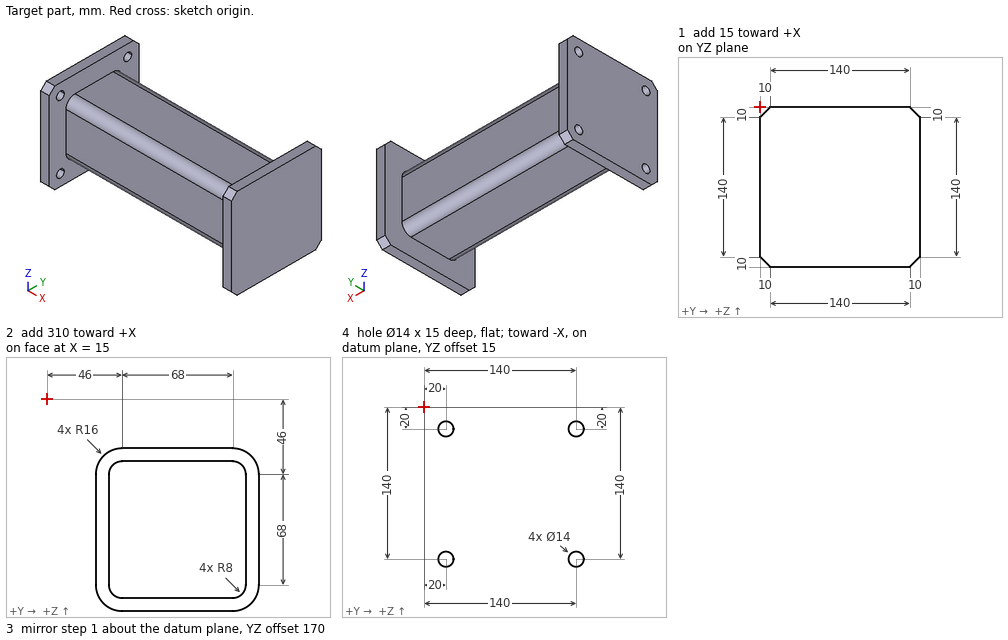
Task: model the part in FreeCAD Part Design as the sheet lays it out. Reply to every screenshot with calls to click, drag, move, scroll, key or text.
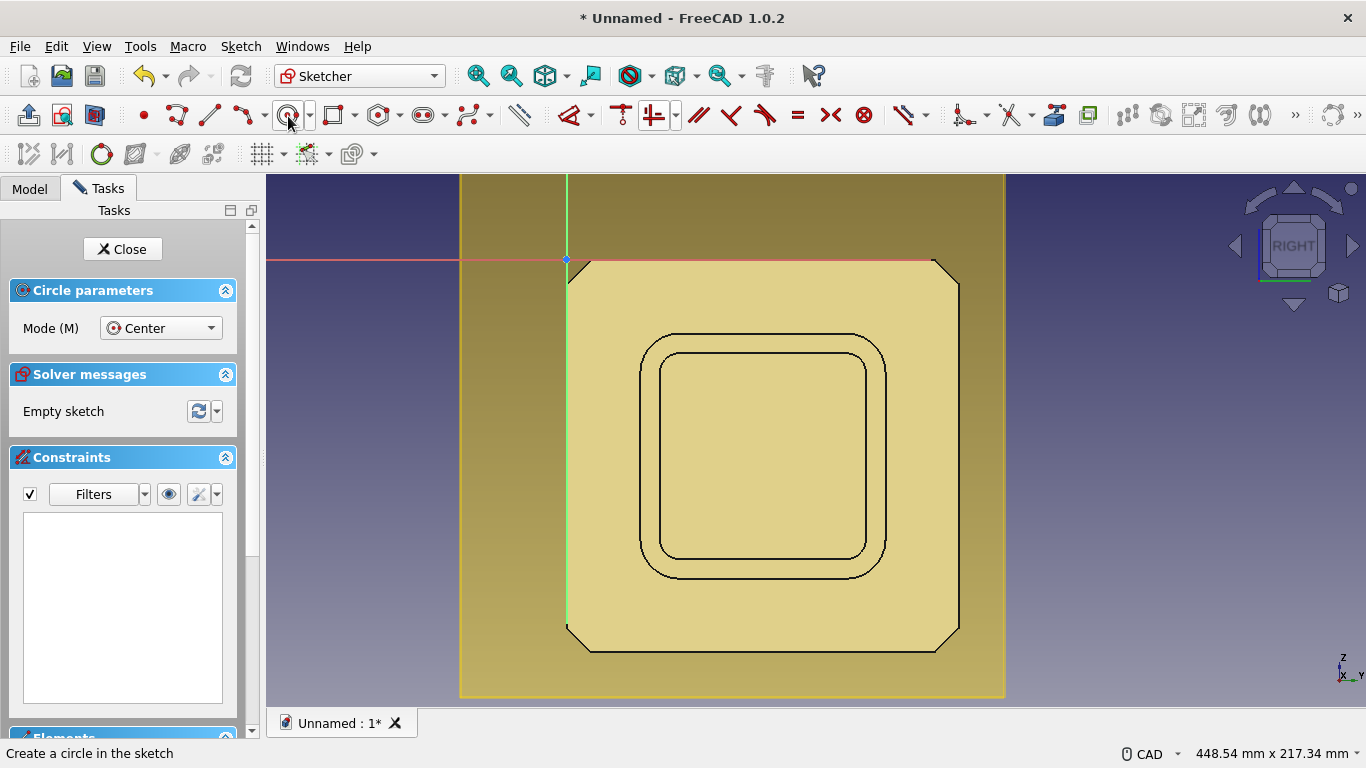
scroll(910, 603, up, 2)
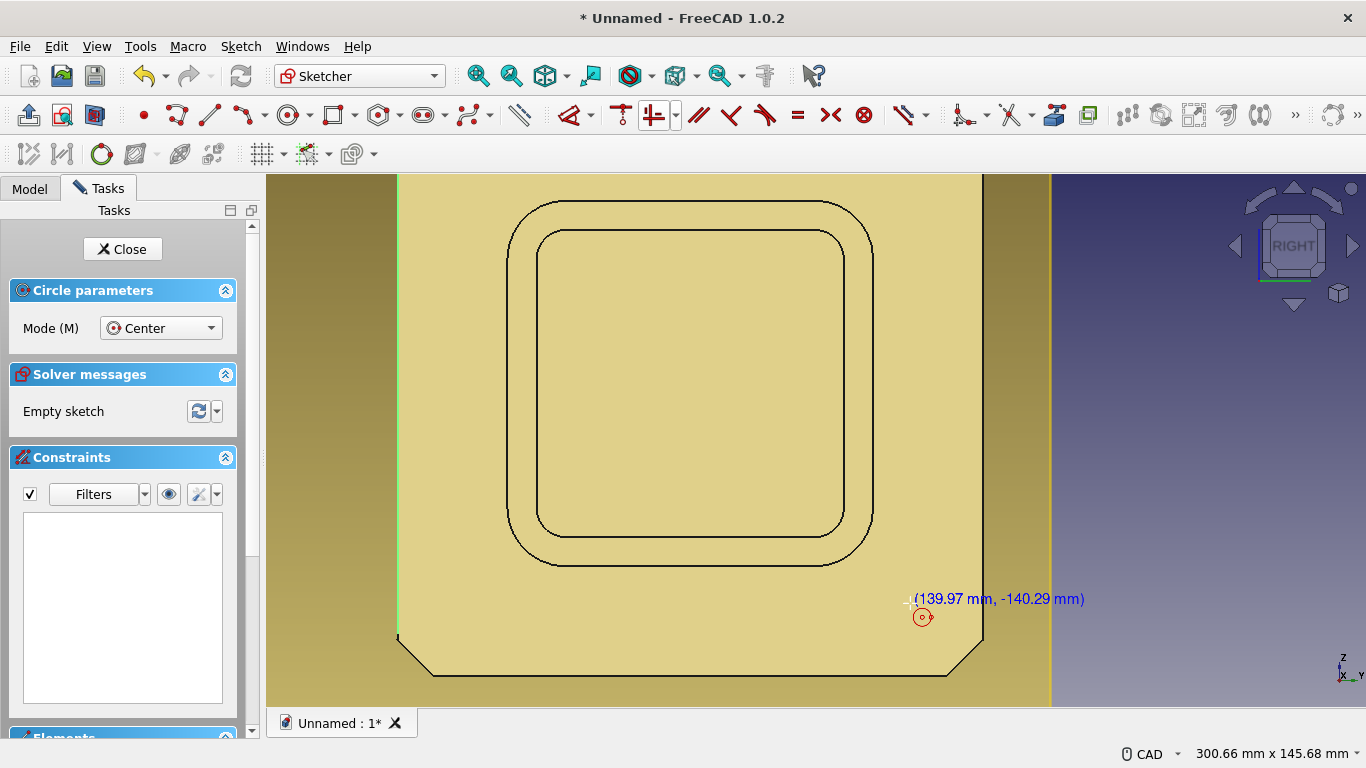
click(910, 603)
move(928, 585)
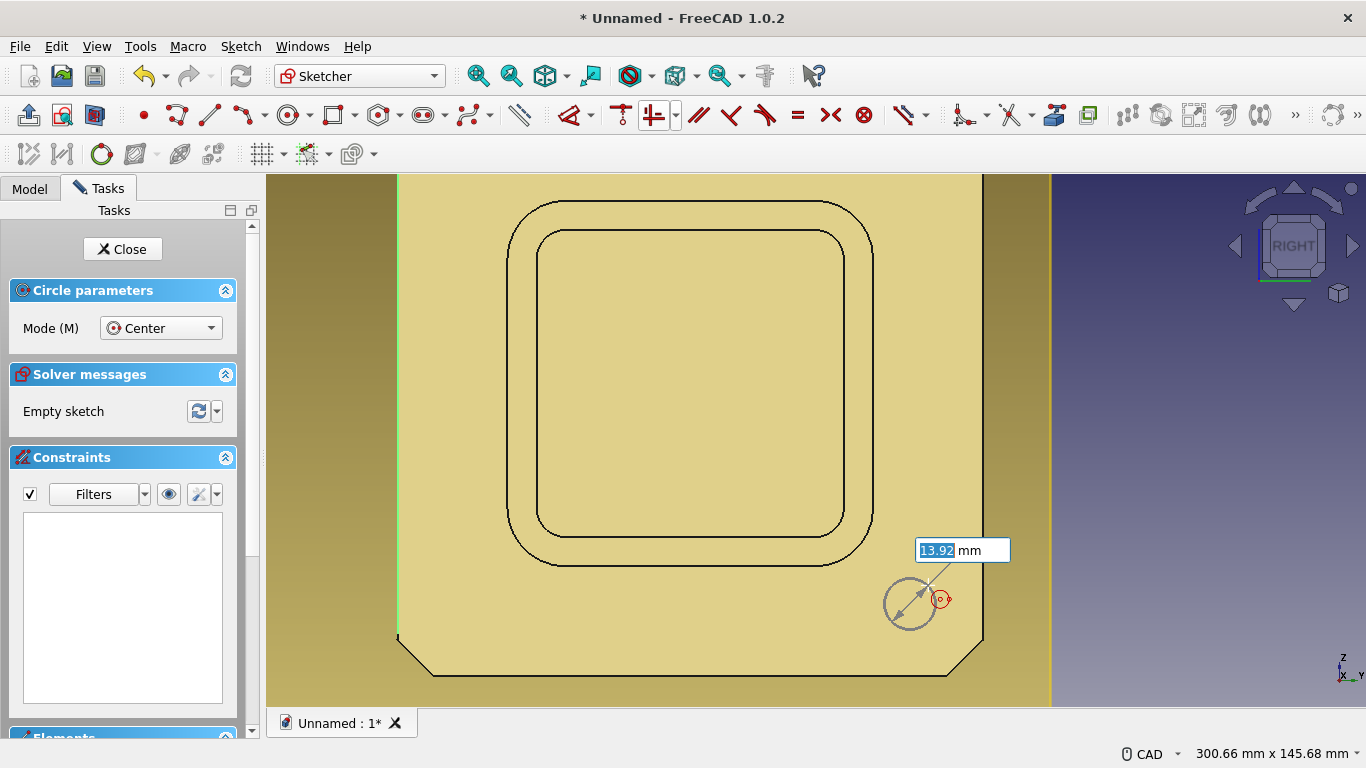
text(14)
key(Return)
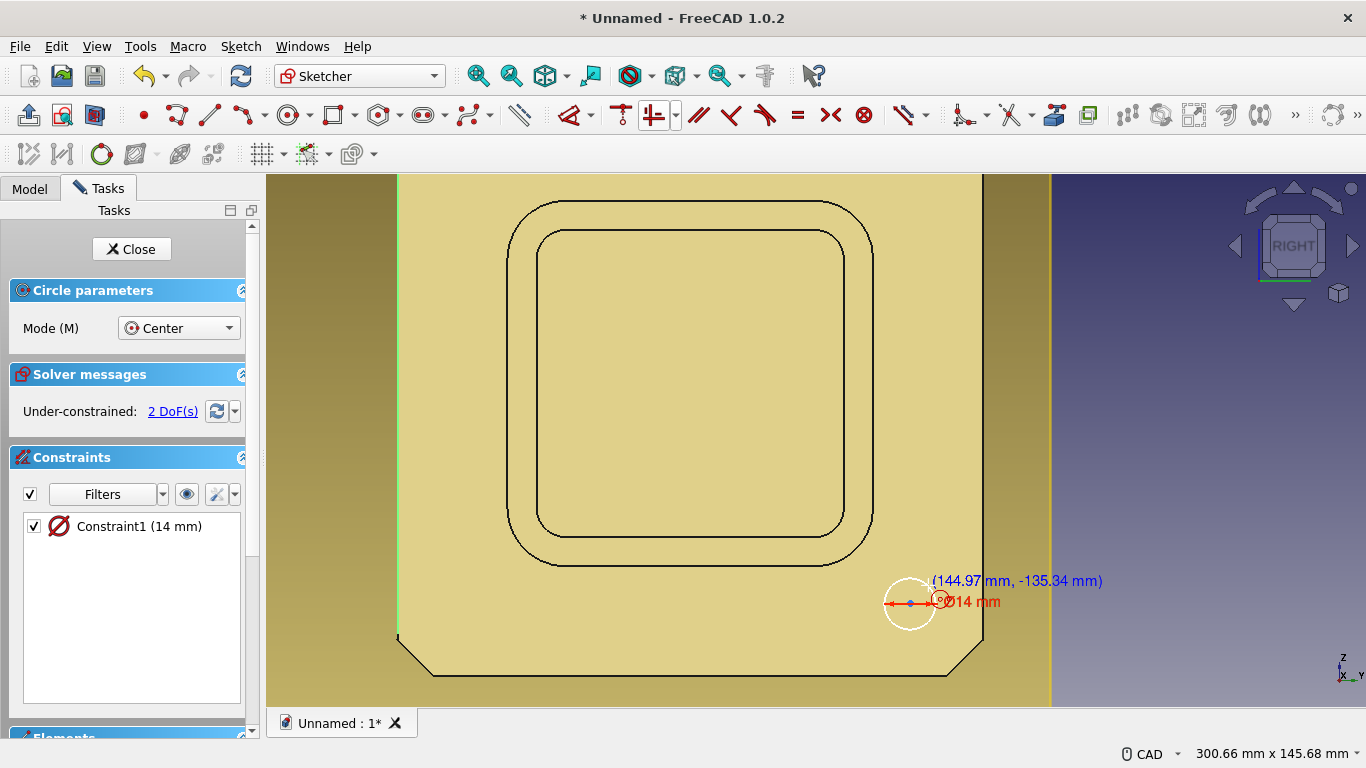
click(471, 603)
move(489, 585)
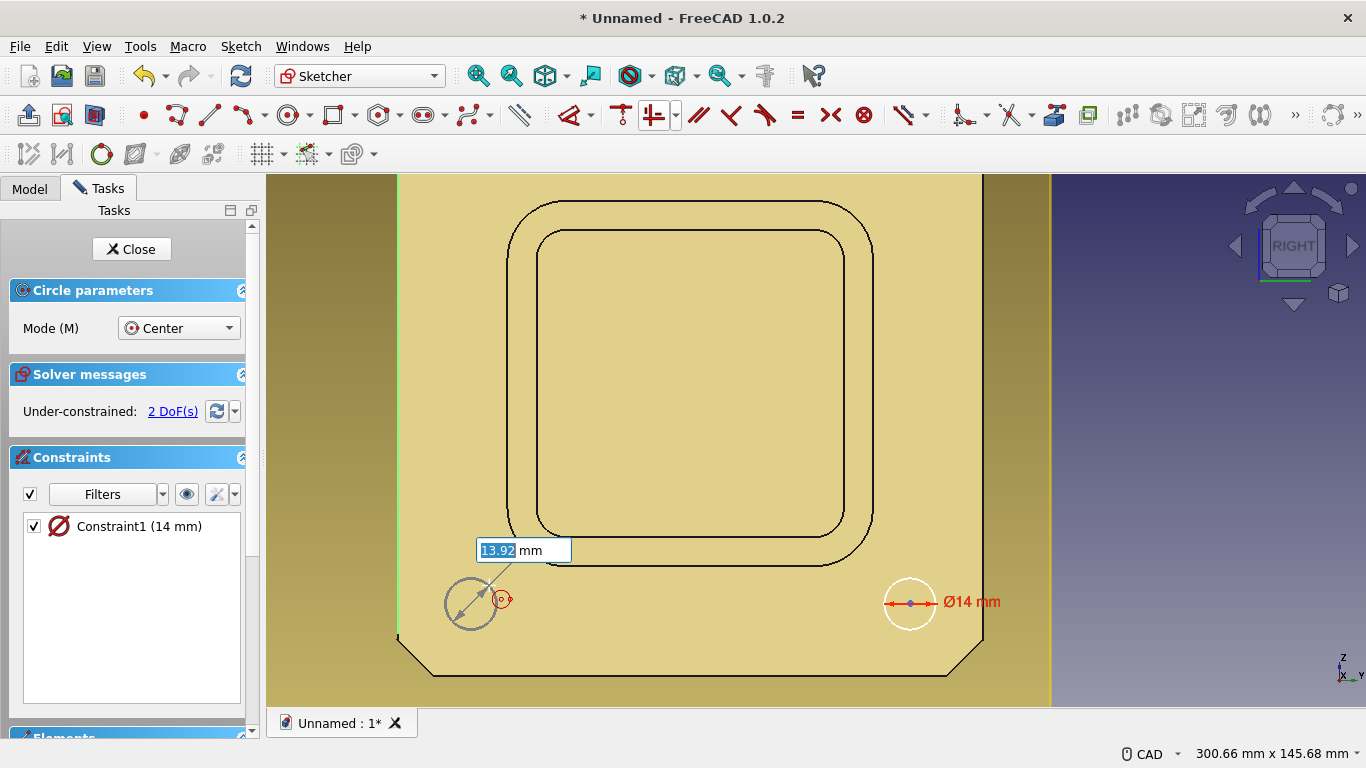
text(14)
key(Return)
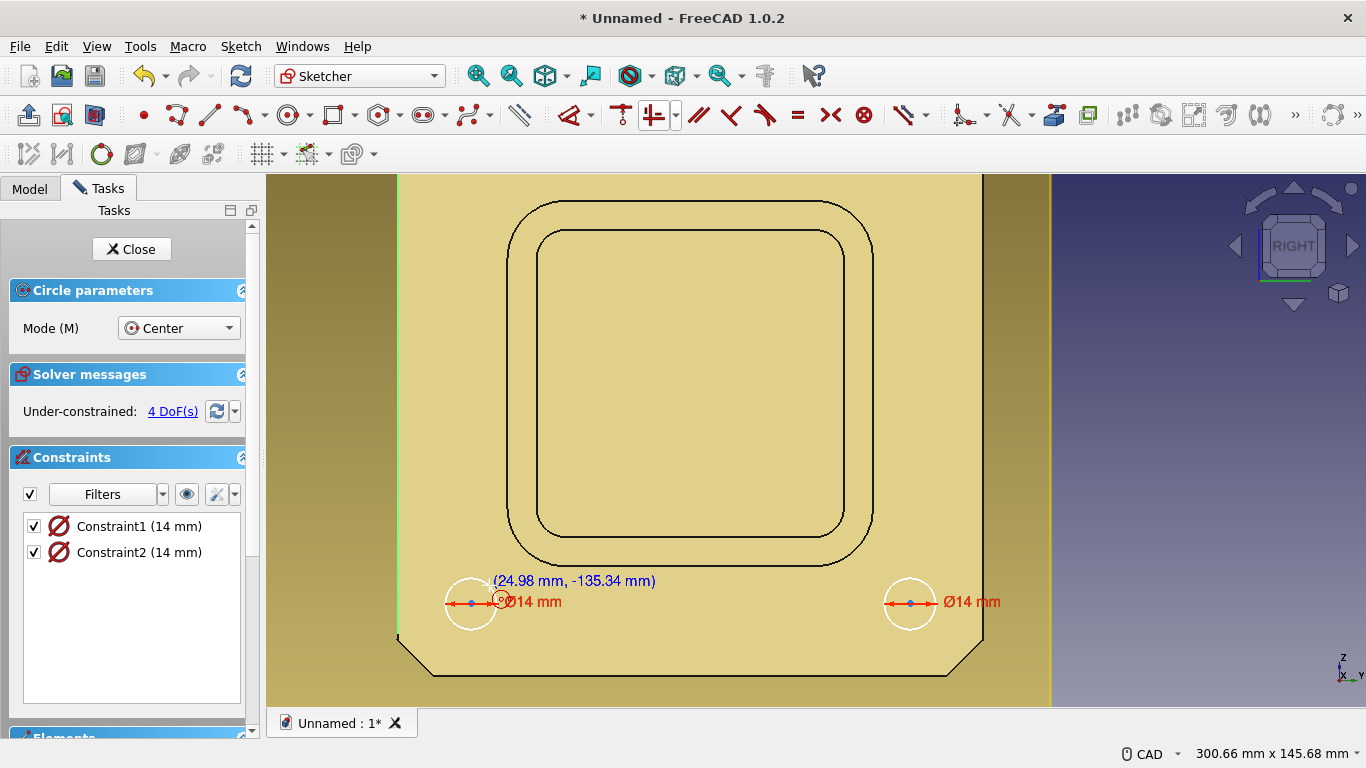
scroll(912, 605, down, 2)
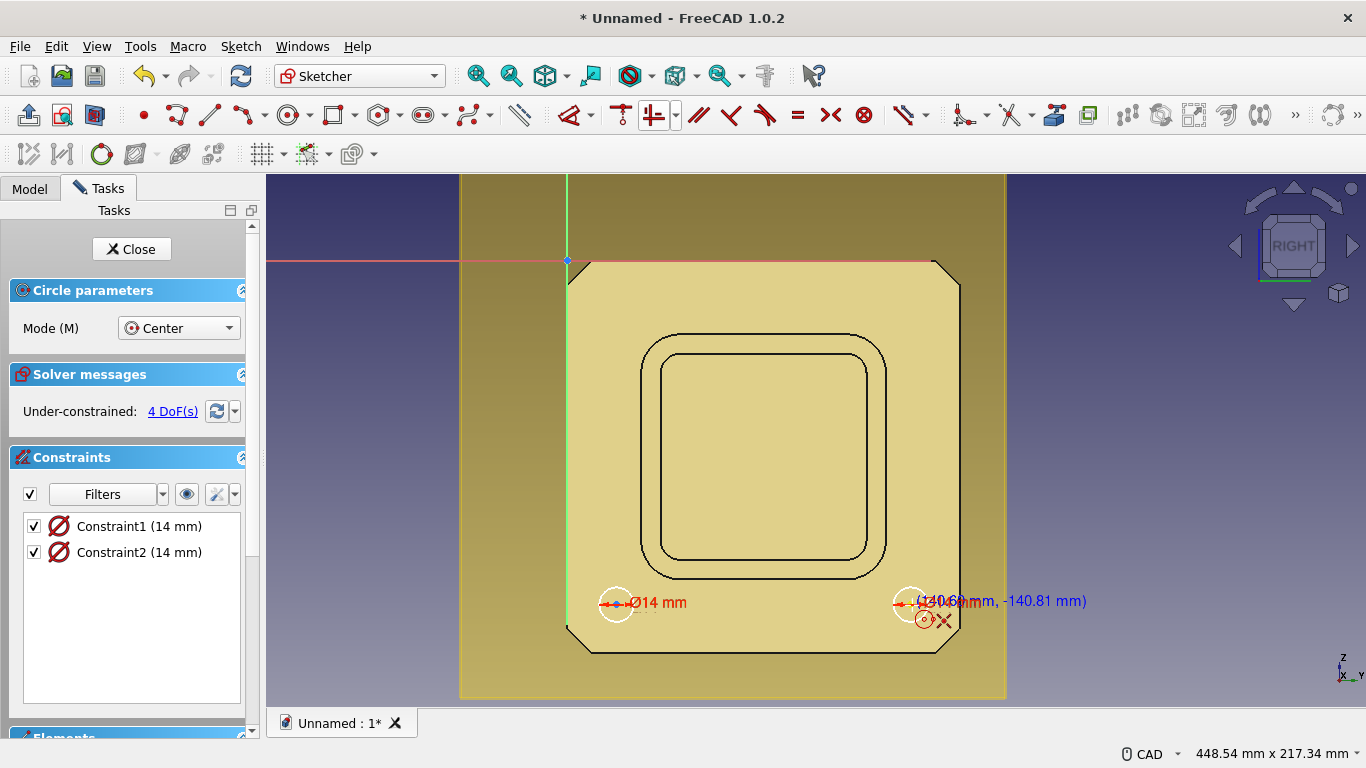
scroll(911, 310, up, 2)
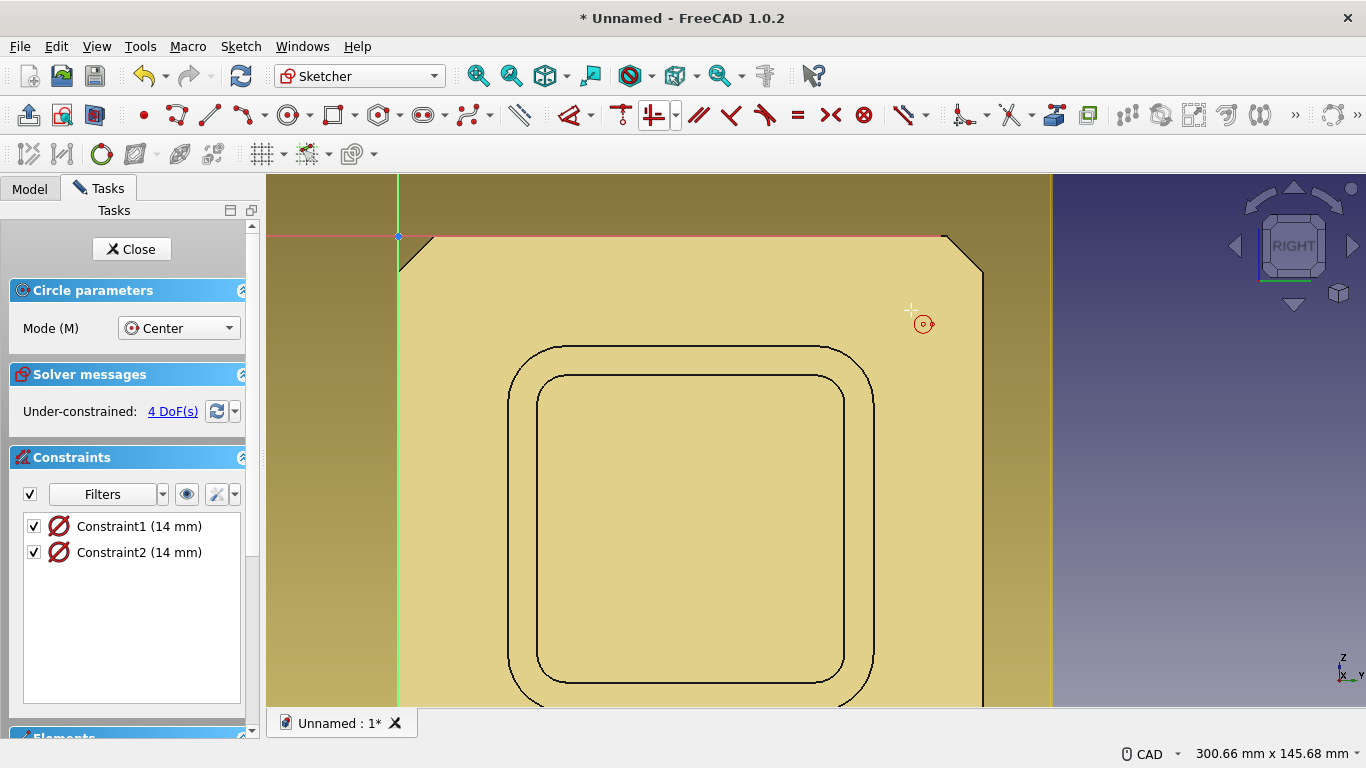
click(910, 309)
move(928, 291)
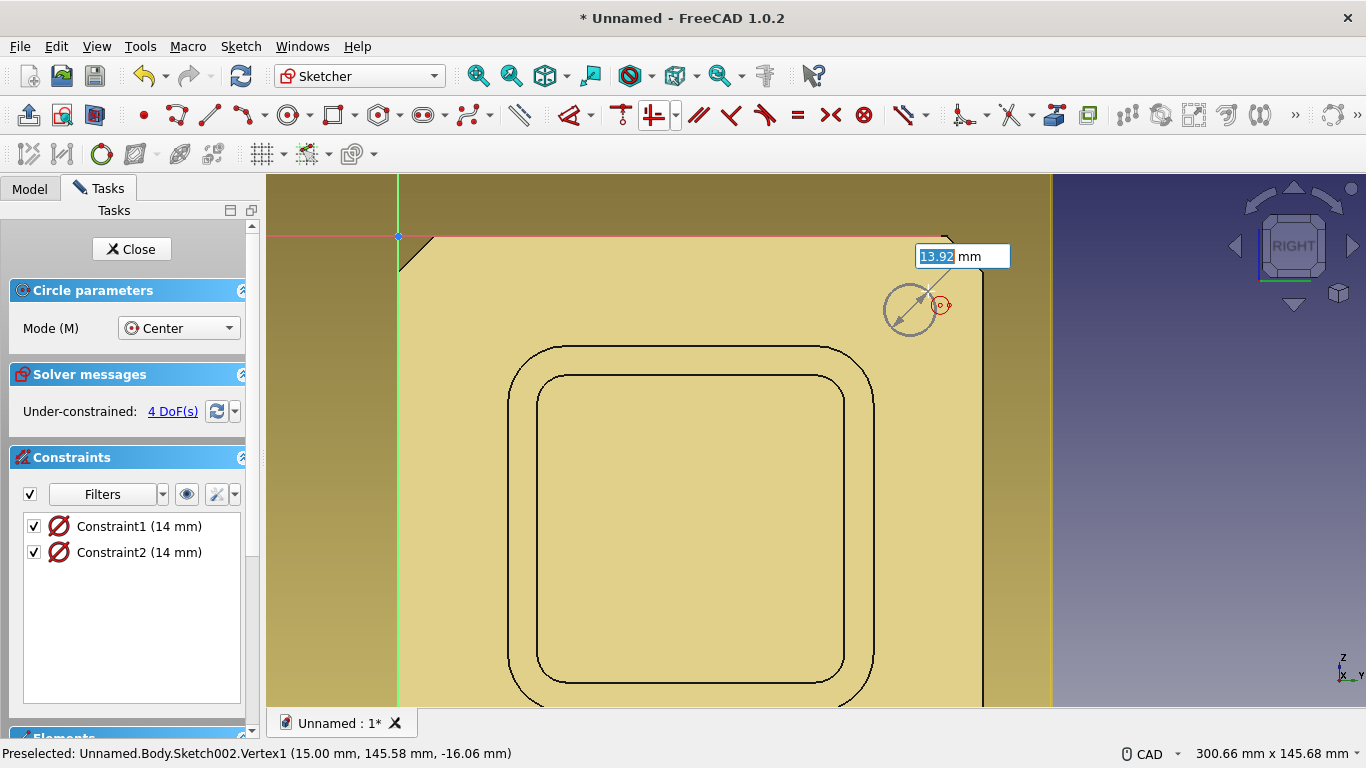
text(14)
key(Return)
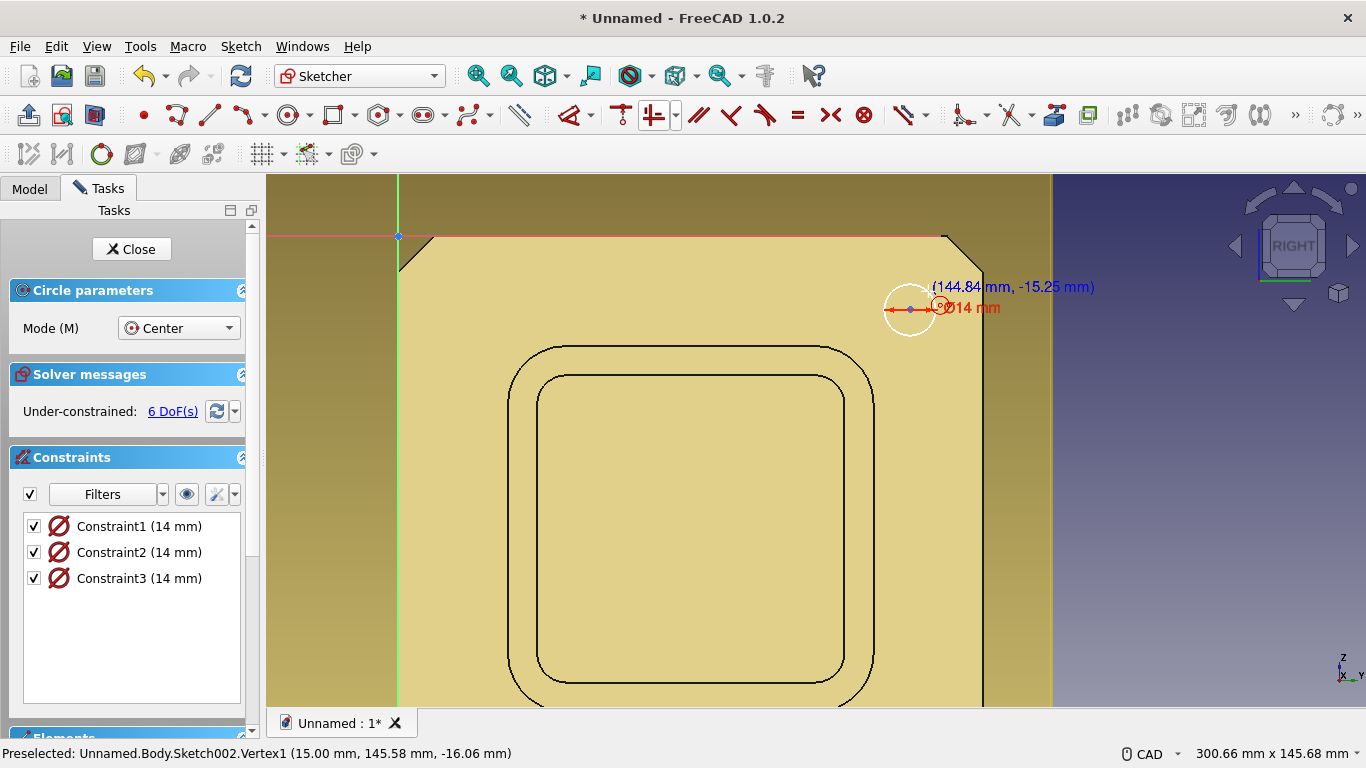
click(471, 309)
move(489, 291)